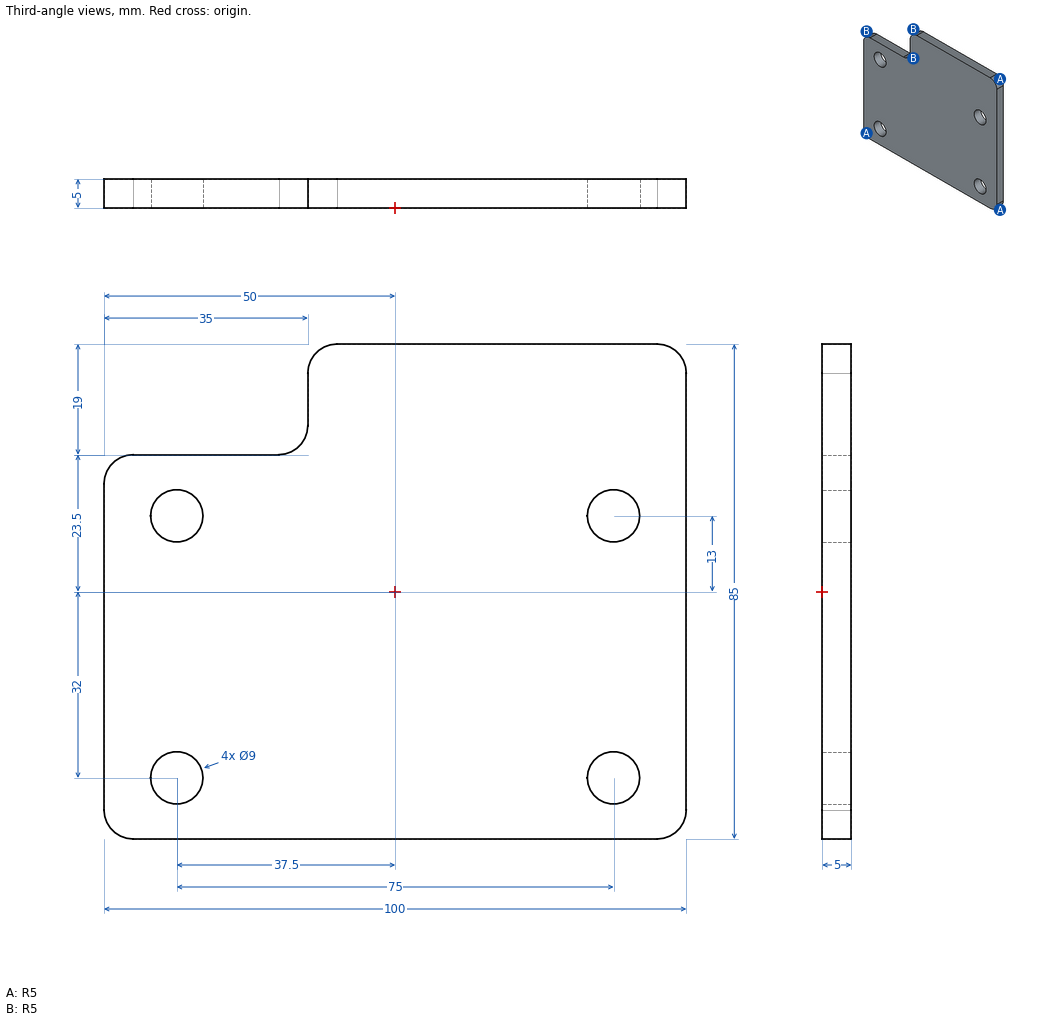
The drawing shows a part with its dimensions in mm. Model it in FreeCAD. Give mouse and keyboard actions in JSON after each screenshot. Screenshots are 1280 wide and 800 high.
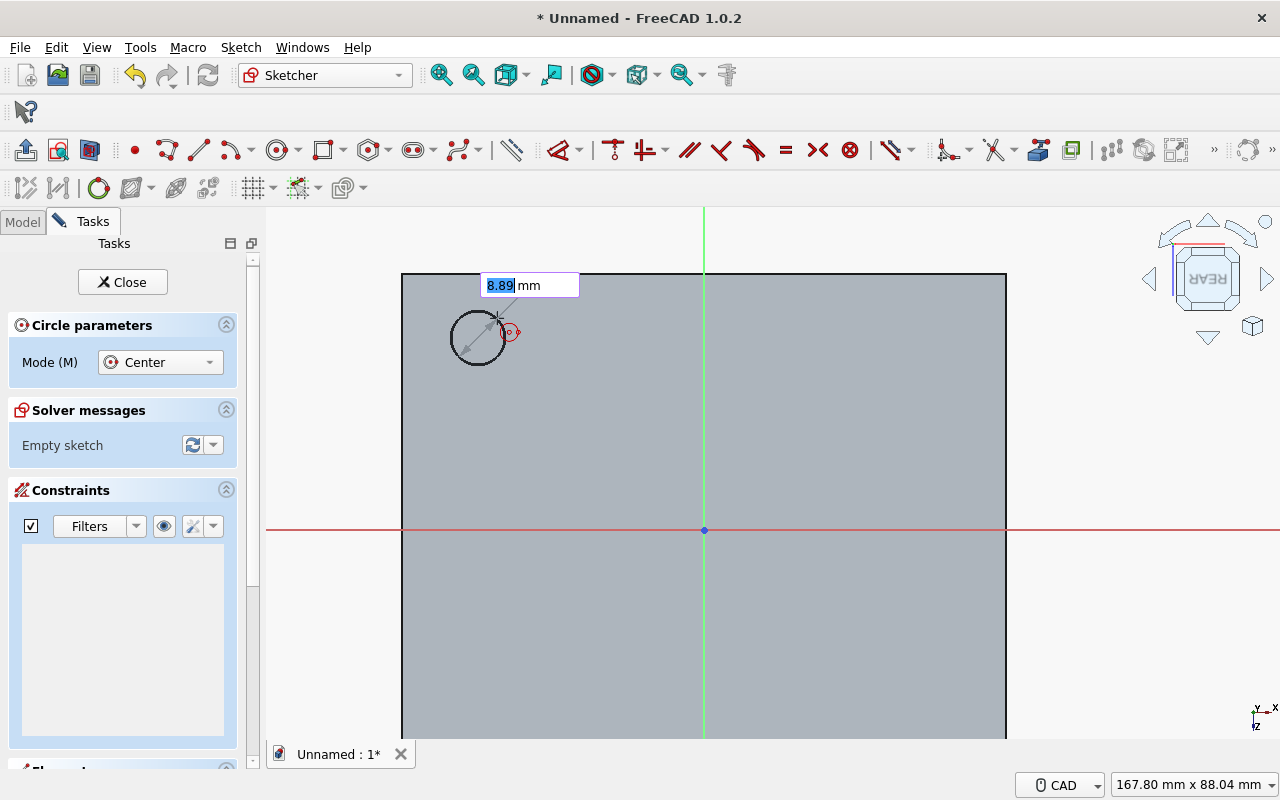
{"action": "type", "text": "9"}
{"action": "key", "text": "Return"}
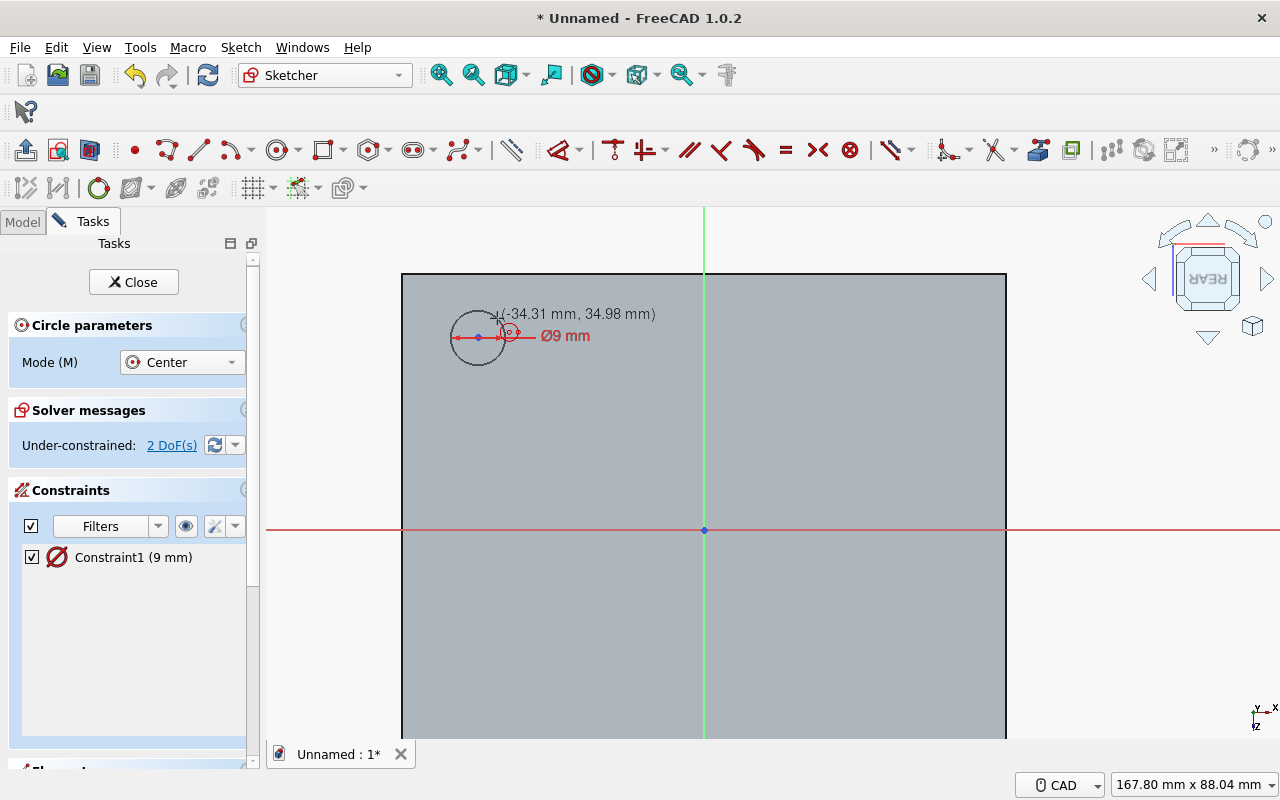
{"action": "left_click", "coordinate": [931, 337]}
{"action": "mouse_move", "coordinate": [950, 318]}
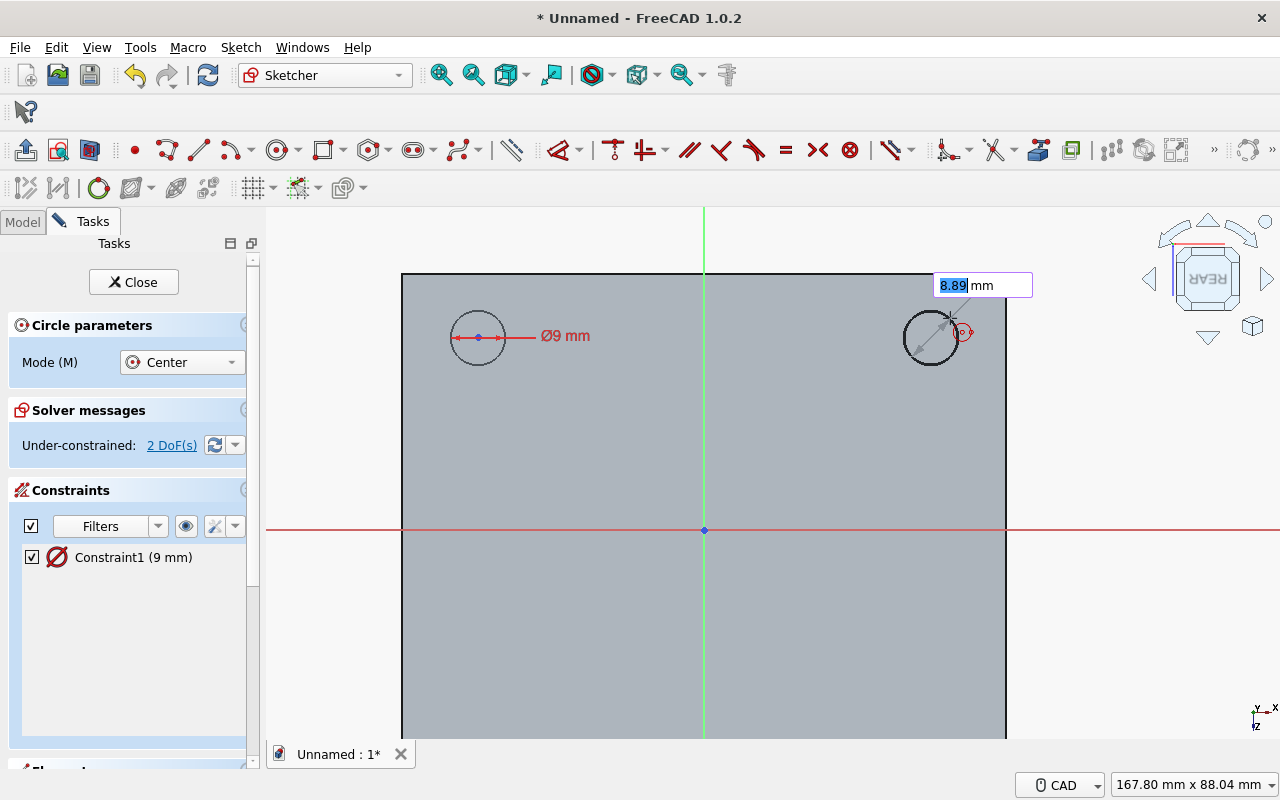
{"action": "type", "text": "9"}
{"action": "key", "text": "Return"}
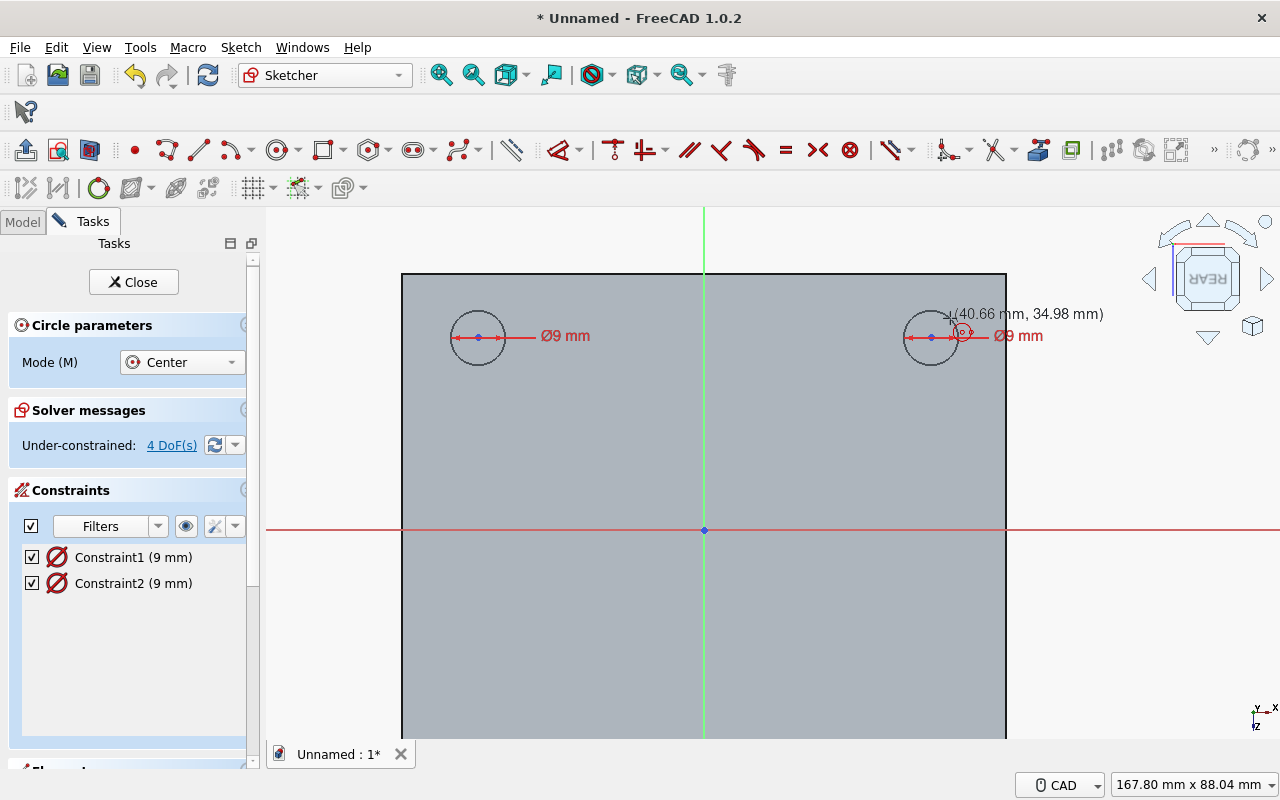
{"action": "left_click", "coordinate": [931, 609]}
{"action": "mouse_move", "coordinate": [950, 590]}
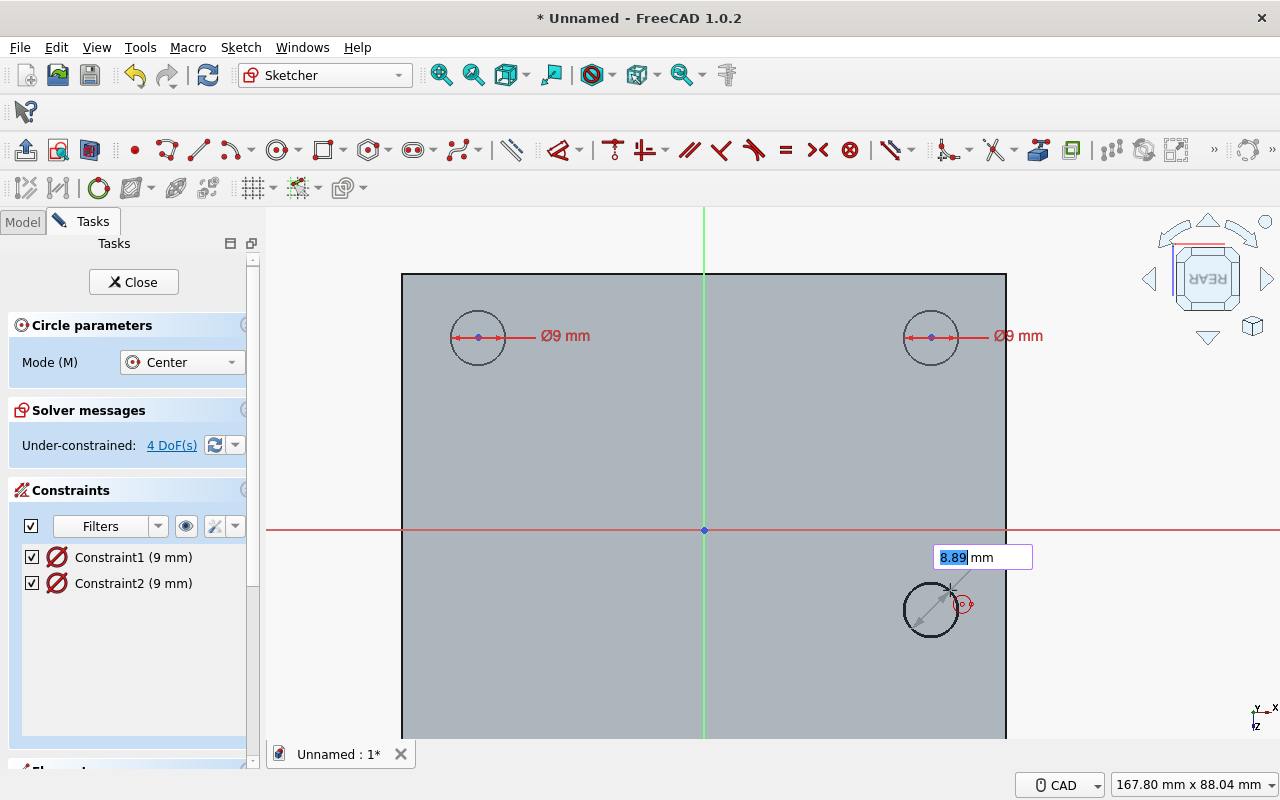
{"action": "type", "text": "9"}
{"action": "key", "text": "Return"}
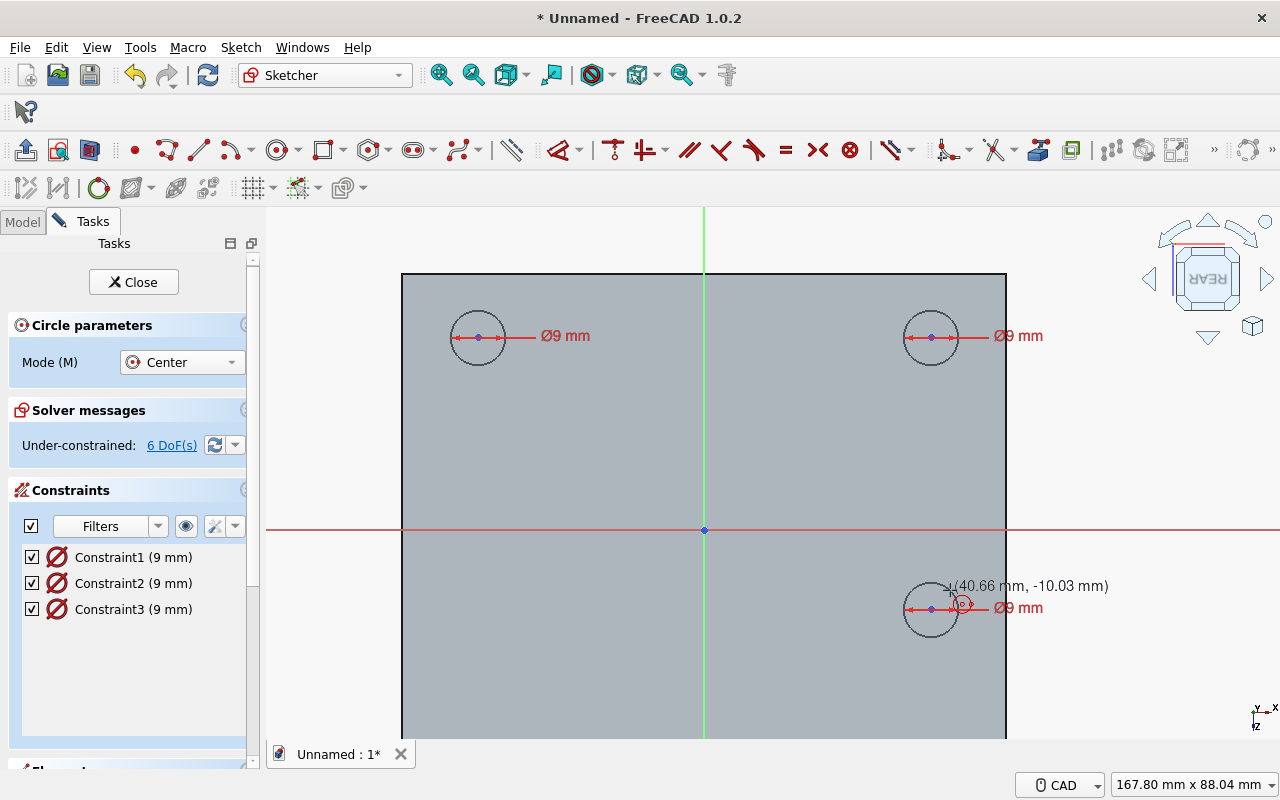
{"action": "left_click", "coordinate": [478, 609]}
{"action": "mouse_move", "coordinate": [497, 590]}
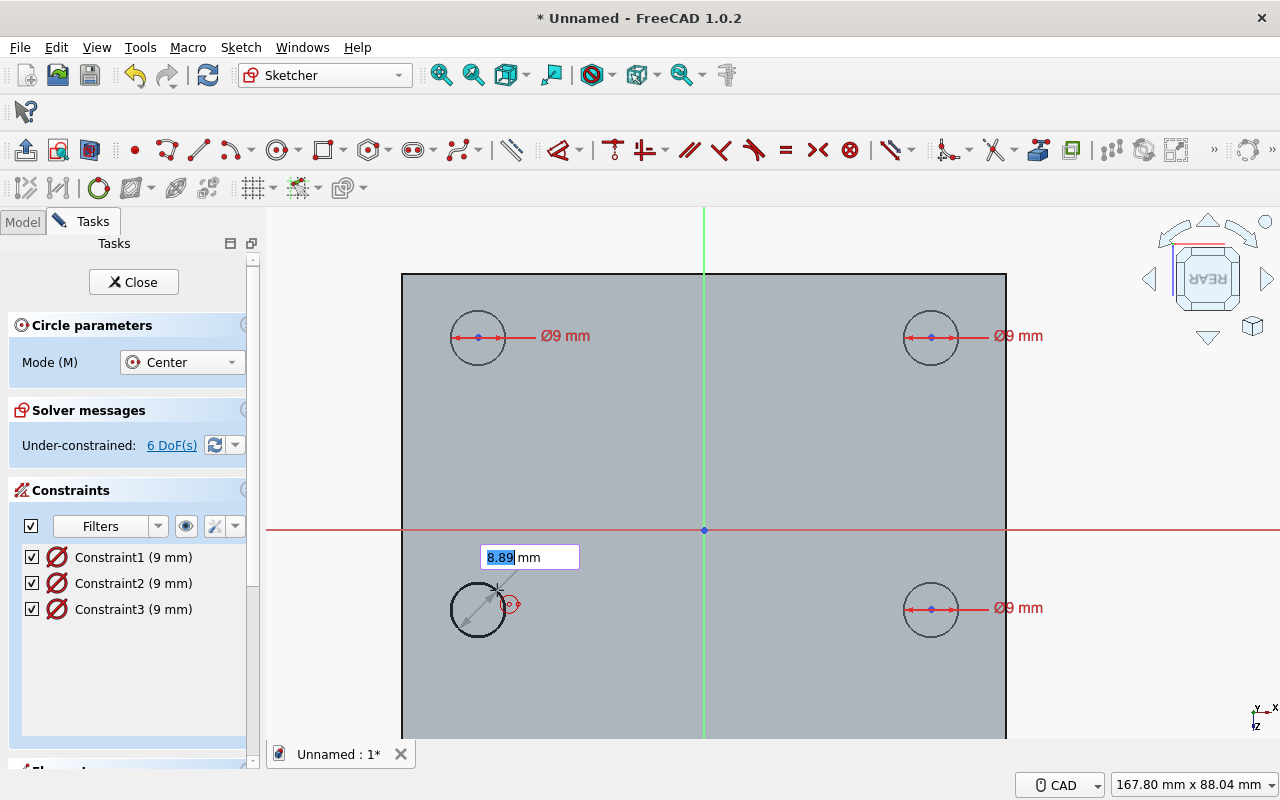
{"action": "type", "text": "9"}
{"action": "key", "text": "Return"}
{"action": "key", "text": "Escape"}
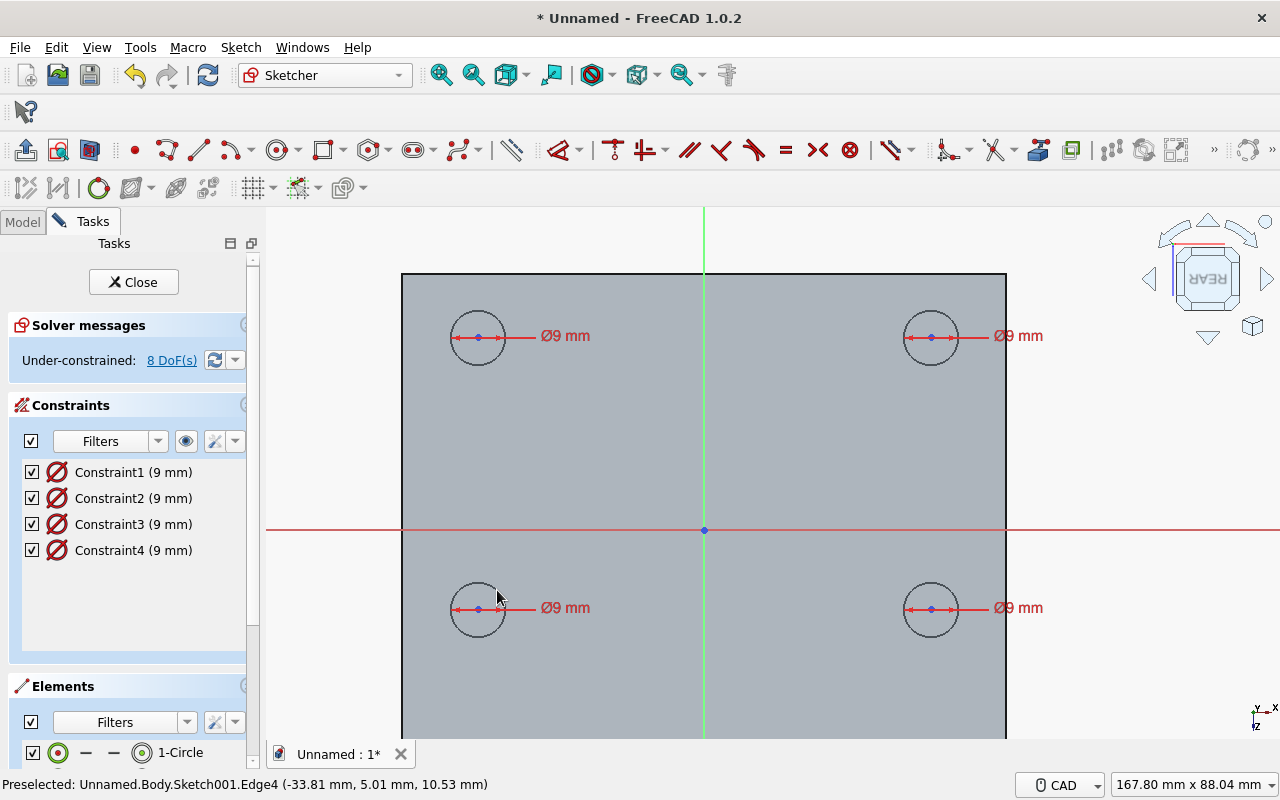
{"action": "left_click", "coordinate": [478, 338]}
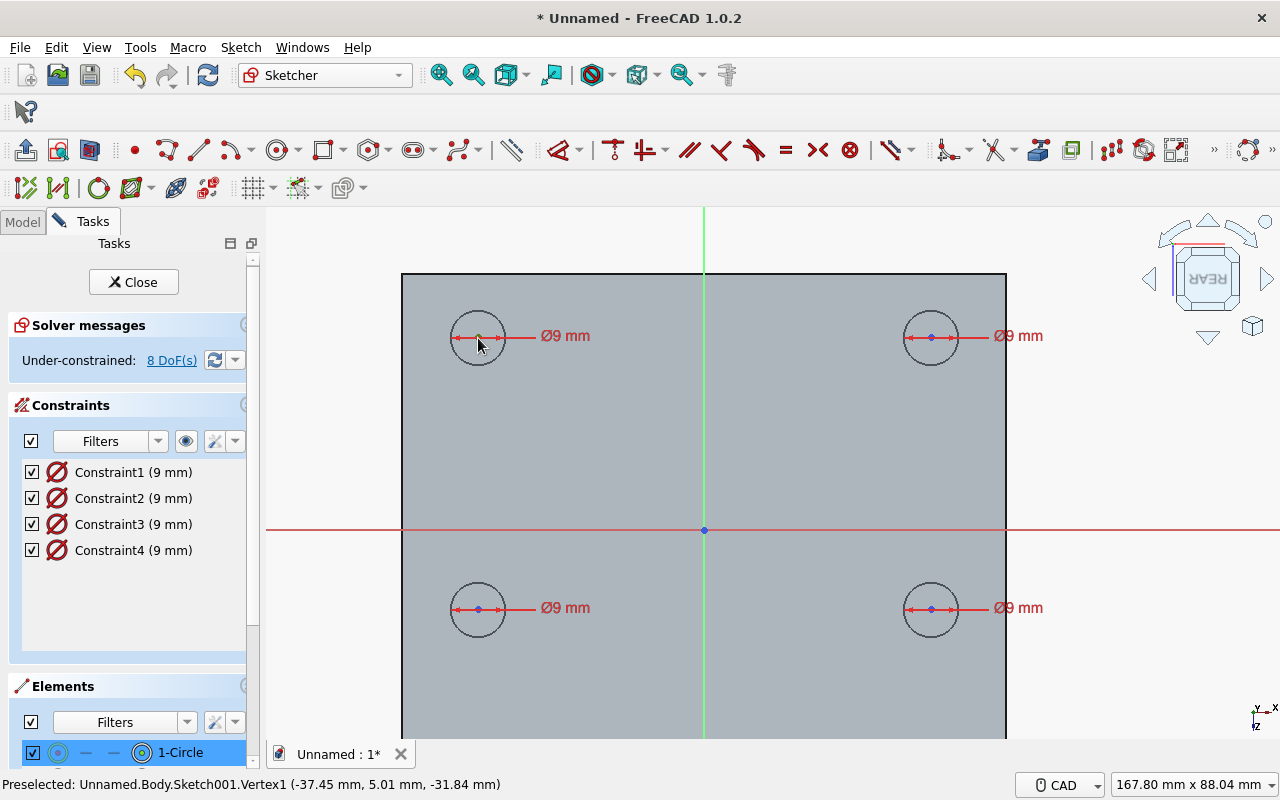
{"action": "left_click", "coordinate": [931, 338]}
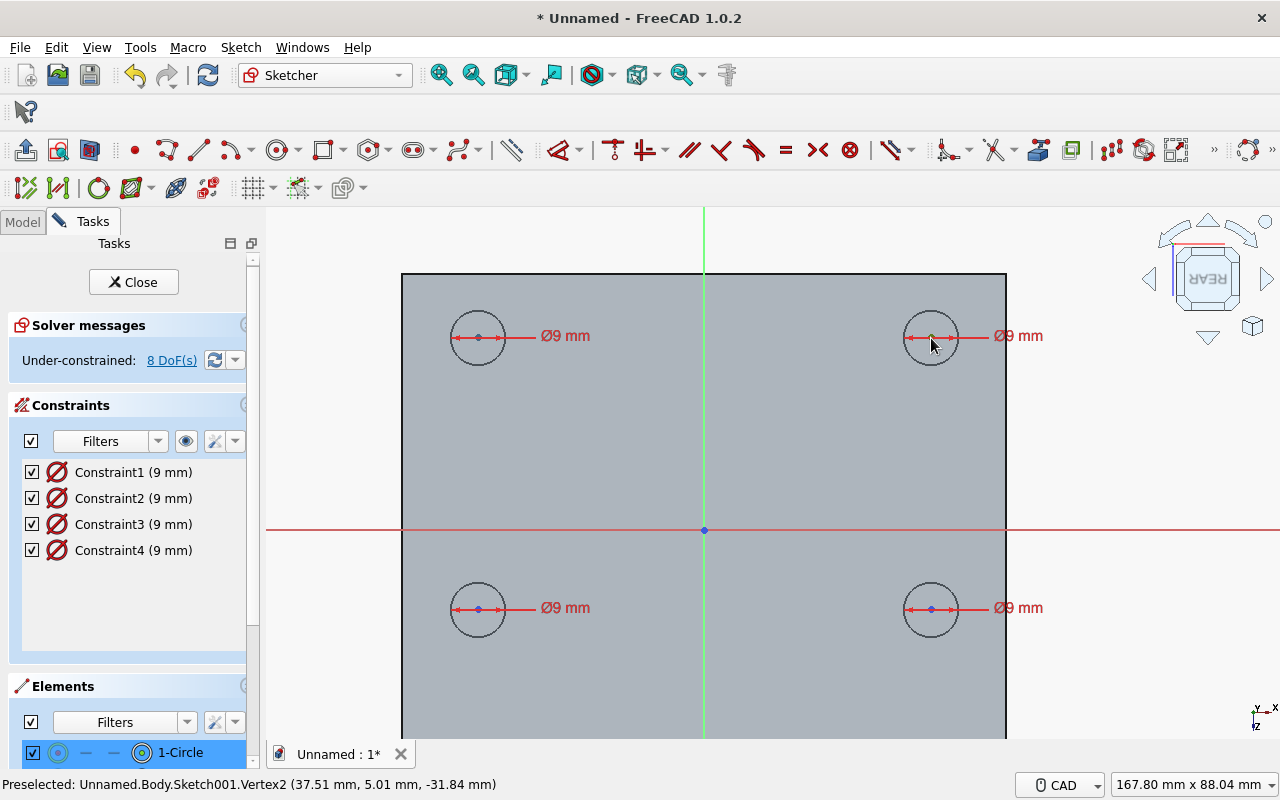
{"action": "left_click", "coordinate": [668, 150]}